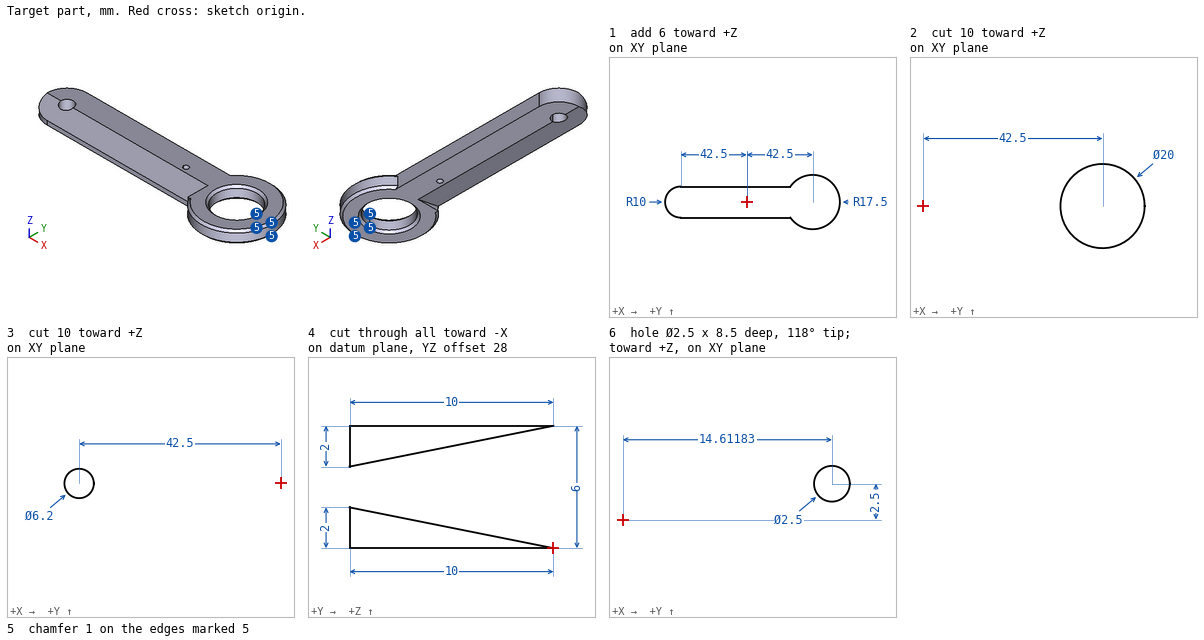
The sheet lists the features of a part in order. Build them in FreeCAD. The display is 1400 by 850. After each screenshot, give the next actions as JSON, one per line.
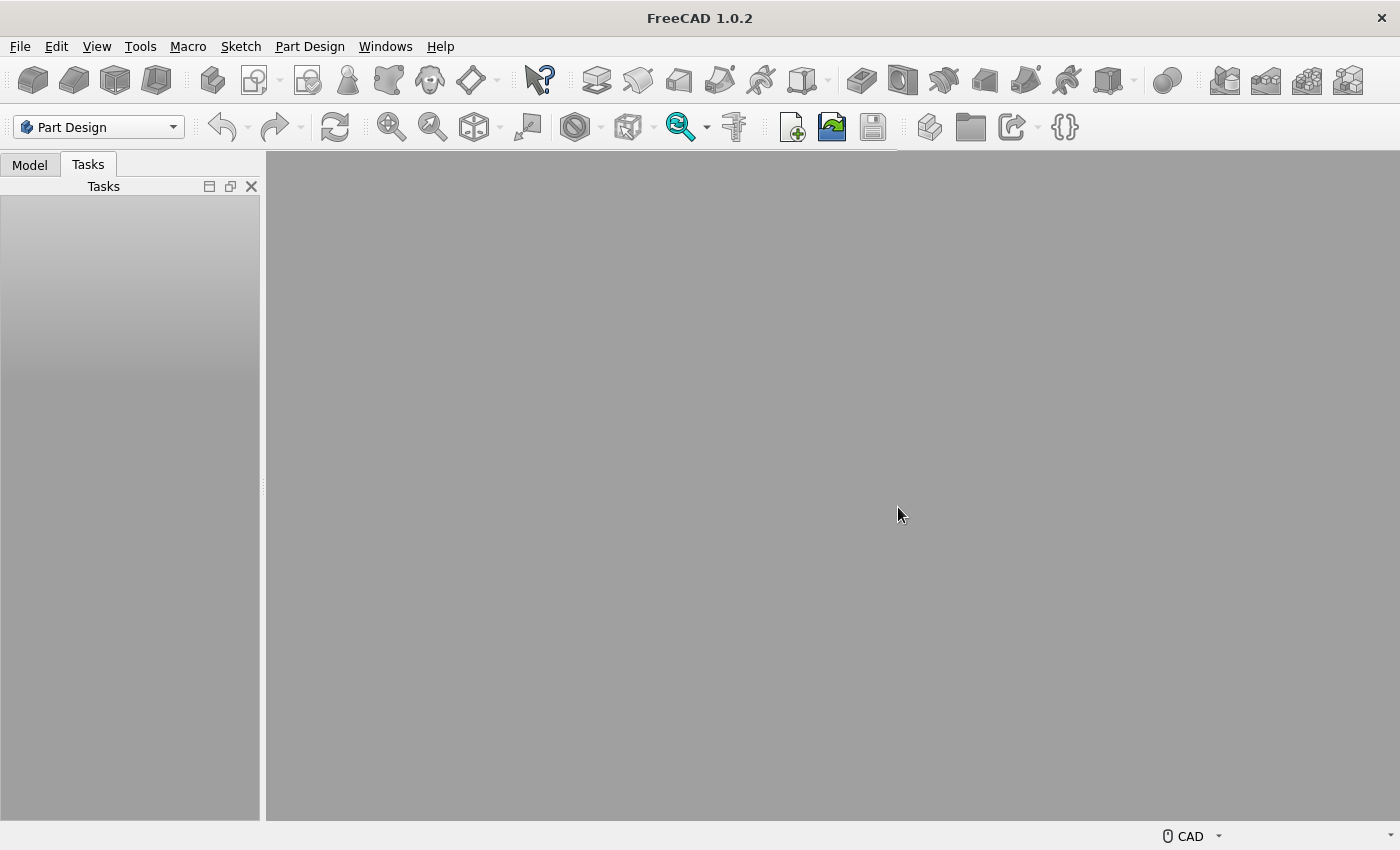
{"action": "key", "text": "ctrl+n"}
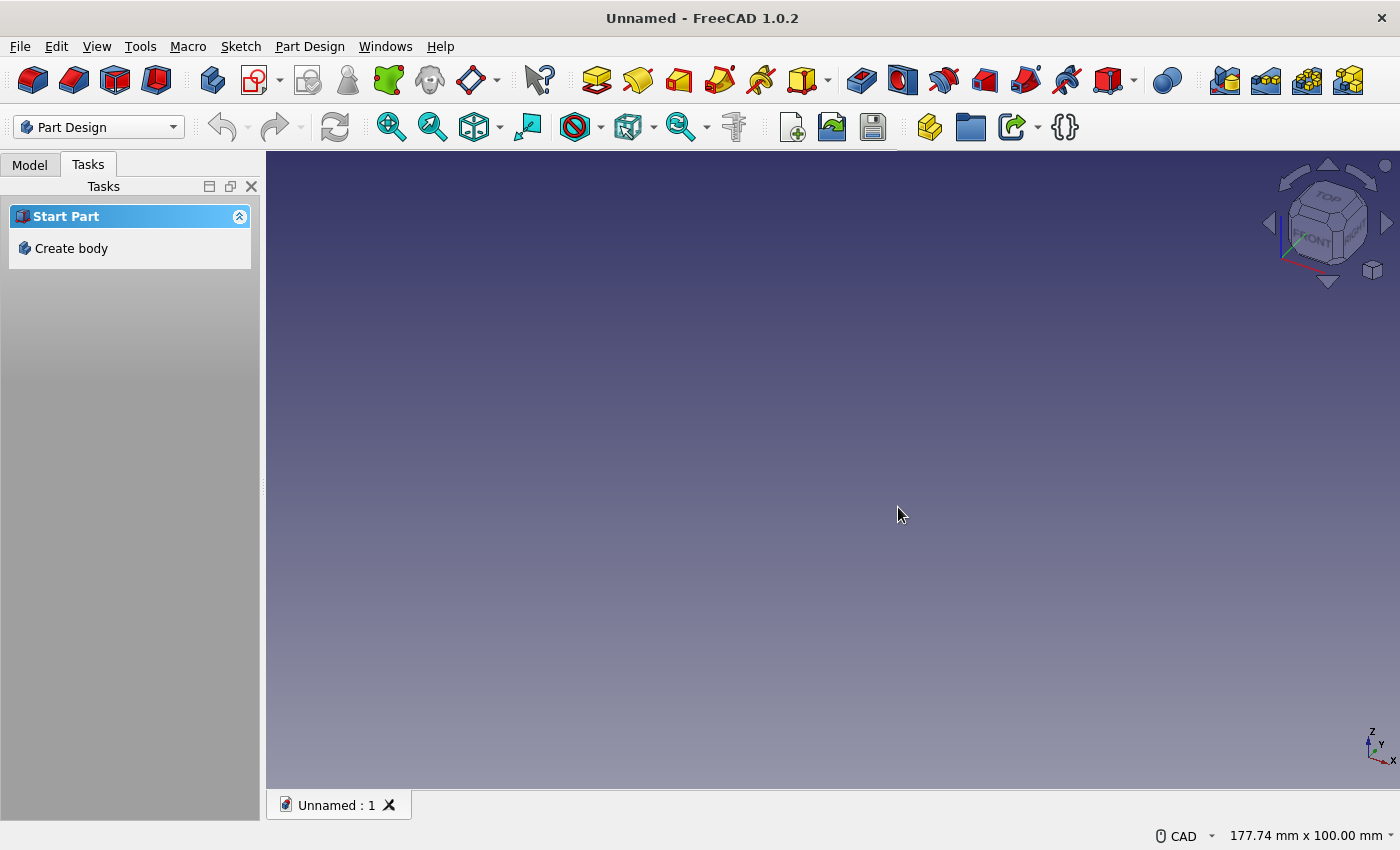
{"action": "left_click", "coordinate": [254, 80]}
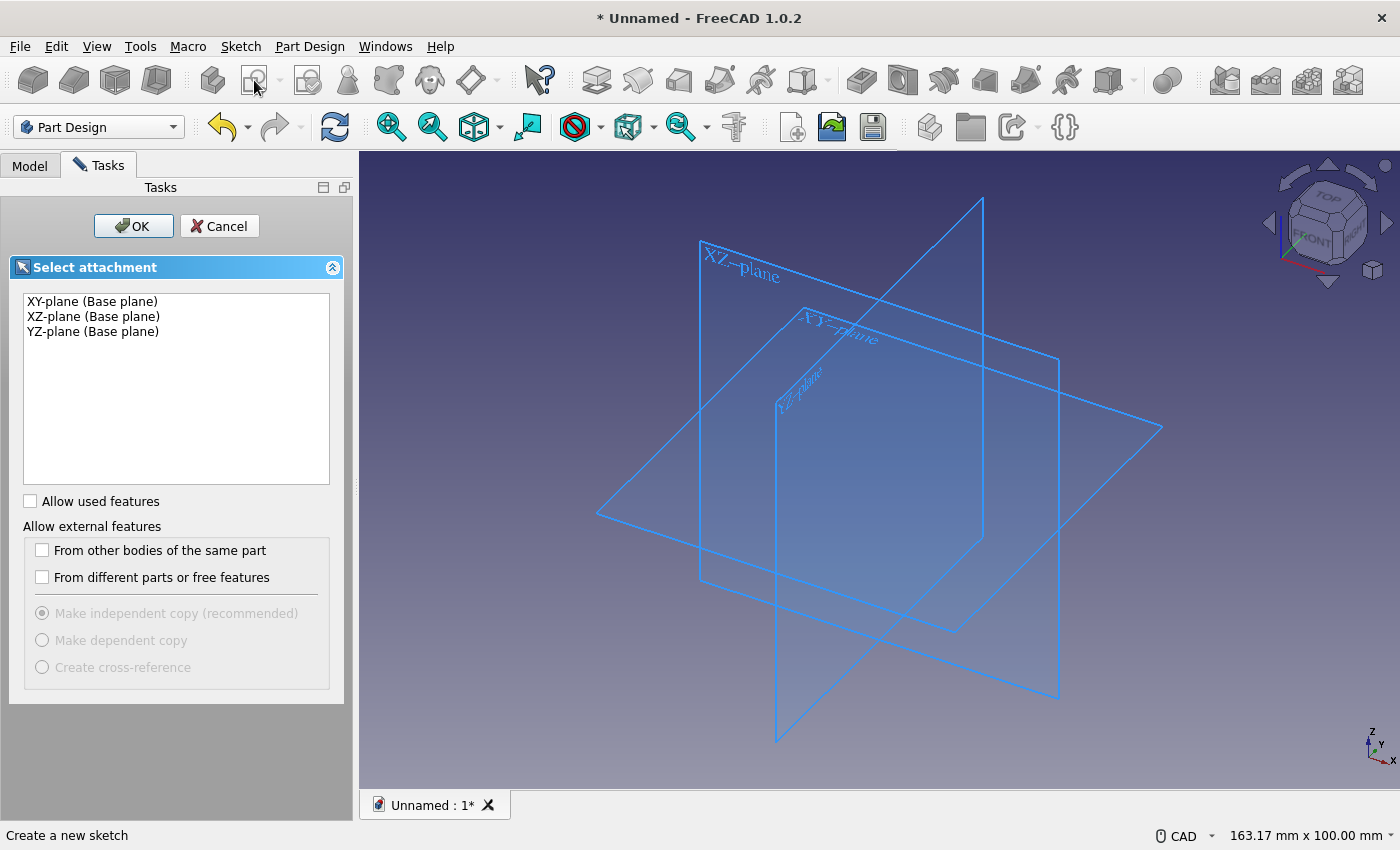
{"action": "left_click", "coordinate": [84, 302]}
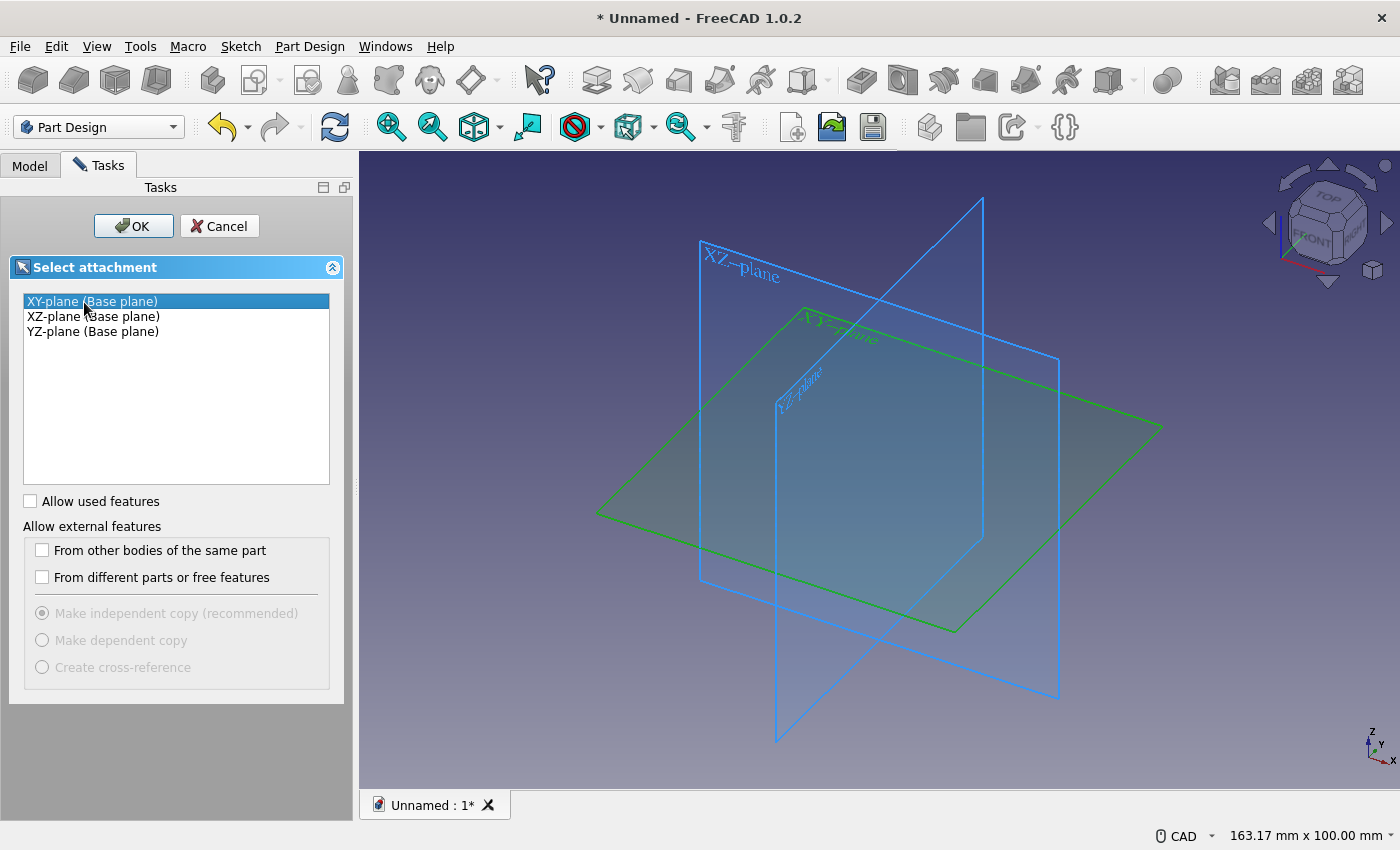
{"action": "left_click", "coordinate": [134, 226]}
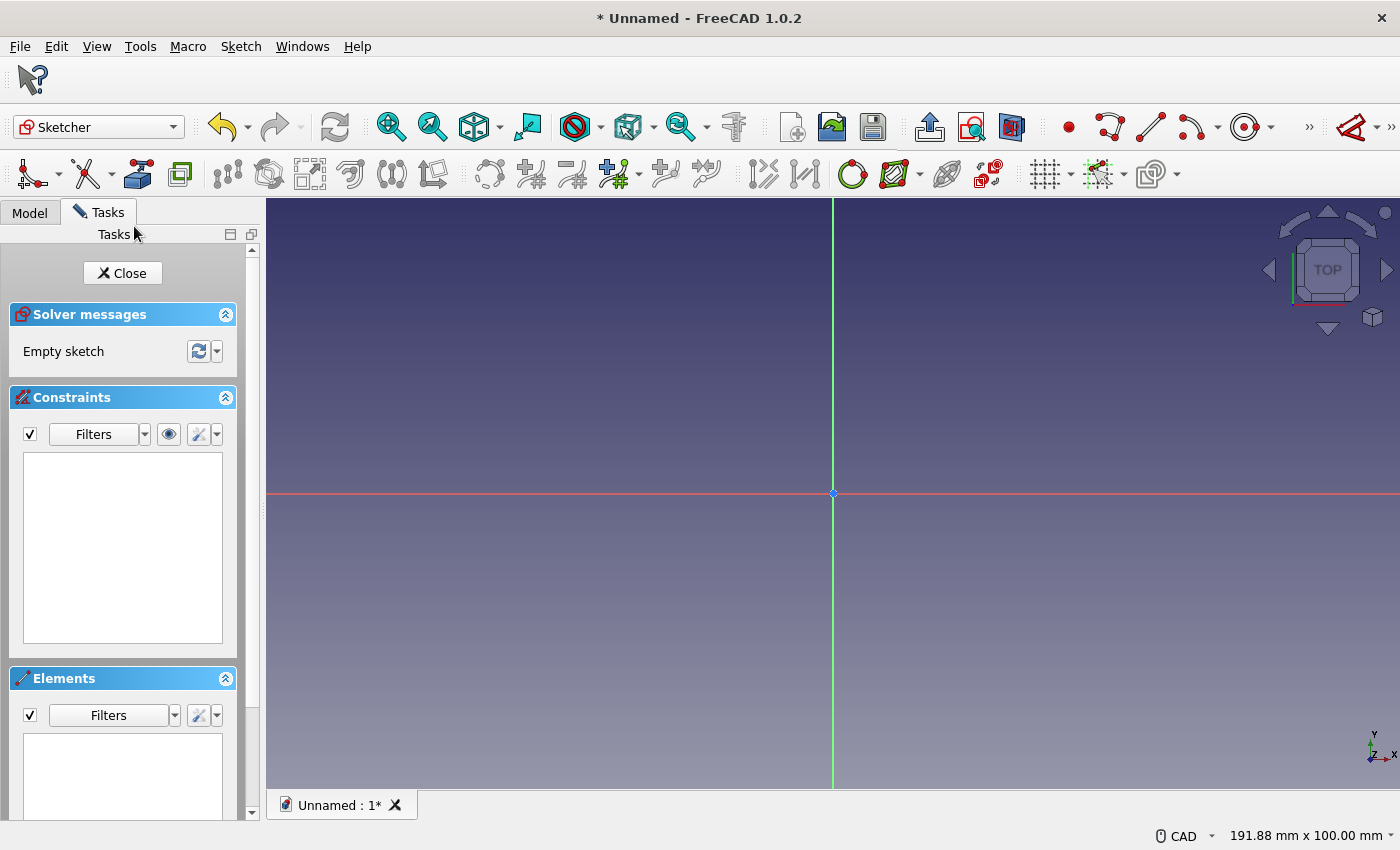
{"action": "key", "text": "g l"}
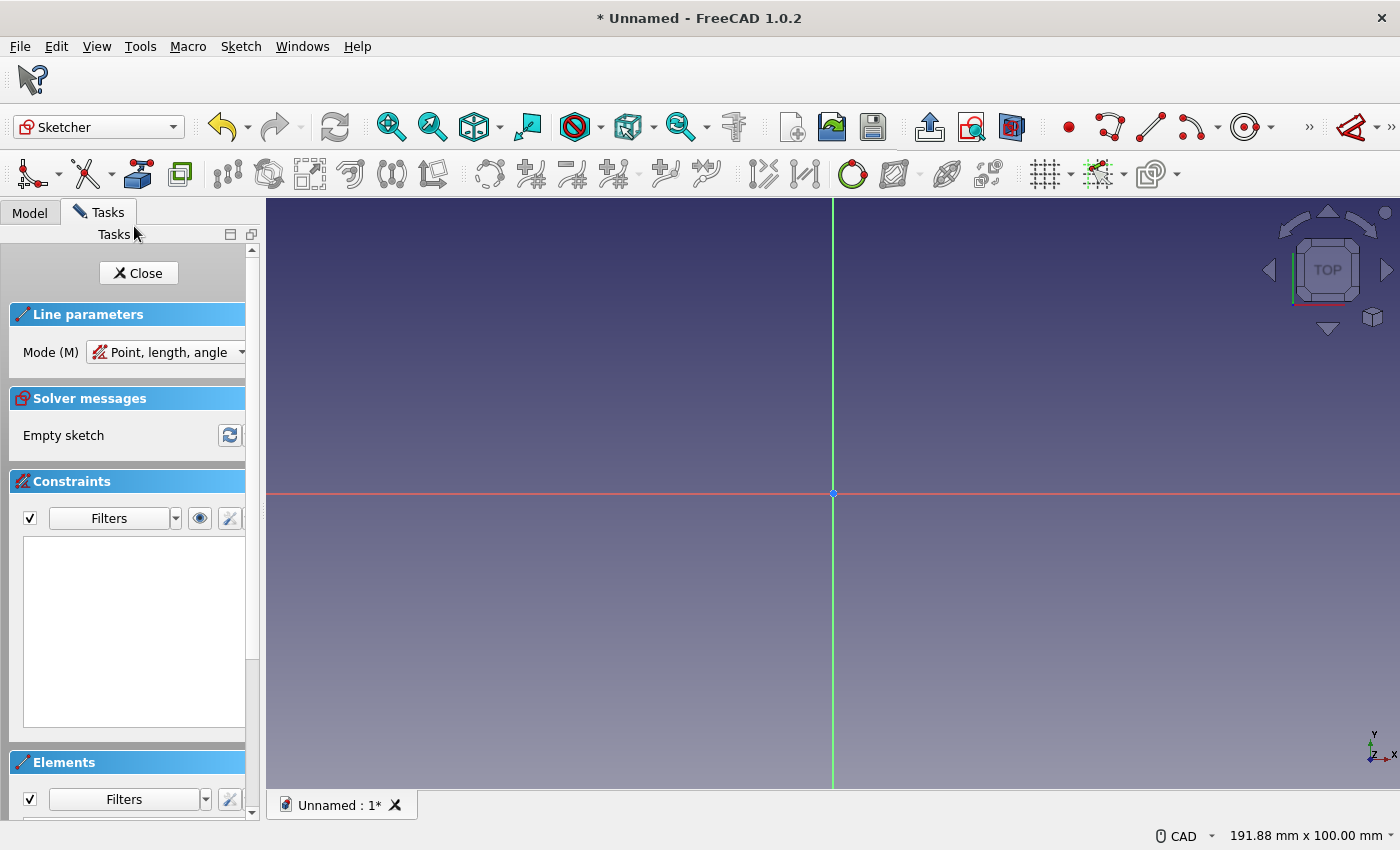
{"action": "left_click", "coordinate": [999, 434]}
{"action": "left_click", "coordinate": [582, 434]}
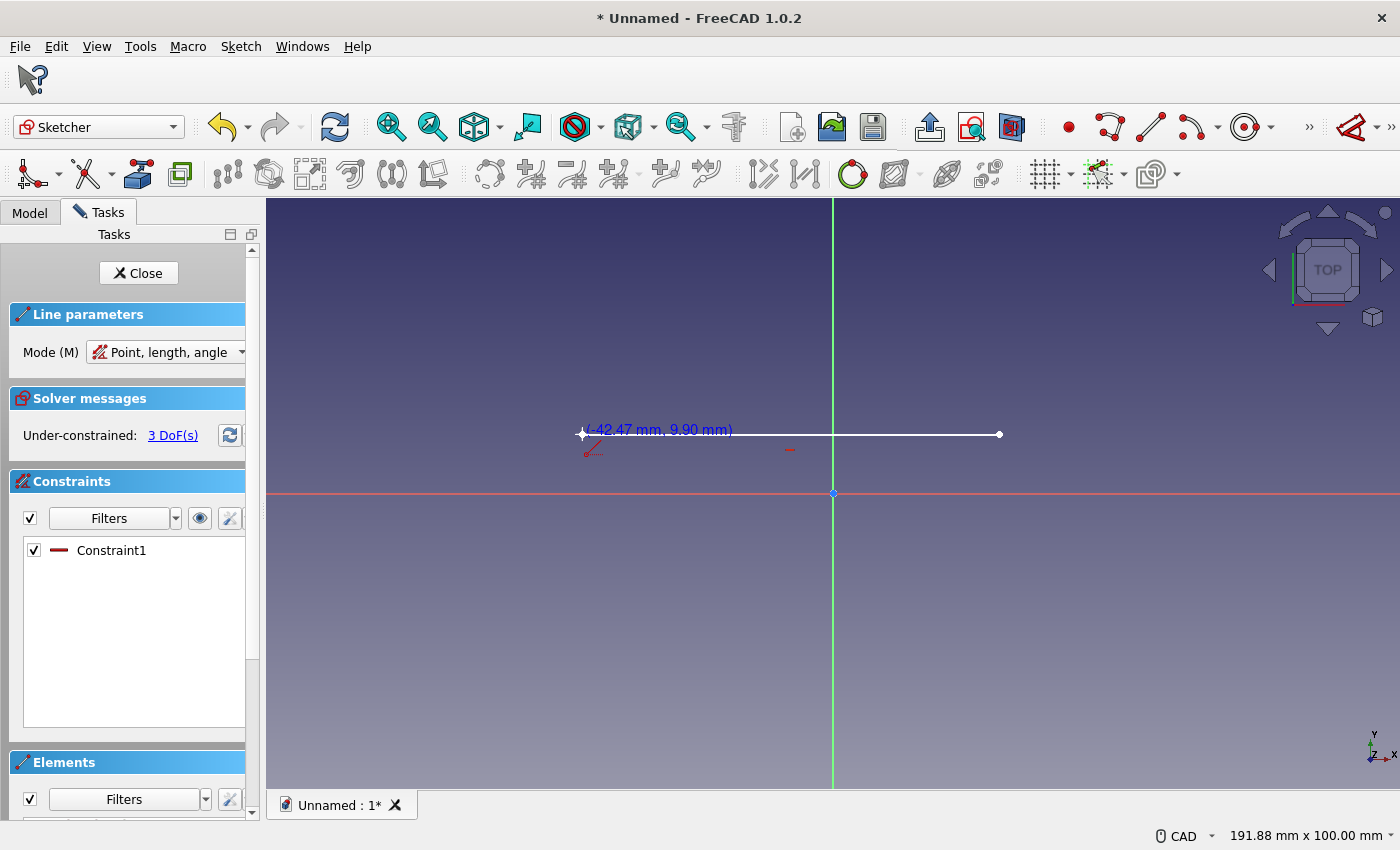
{"action": "left_click", "coordinate": [582, 553]}
{"action": "left_click", "coordinate": [999, 553]}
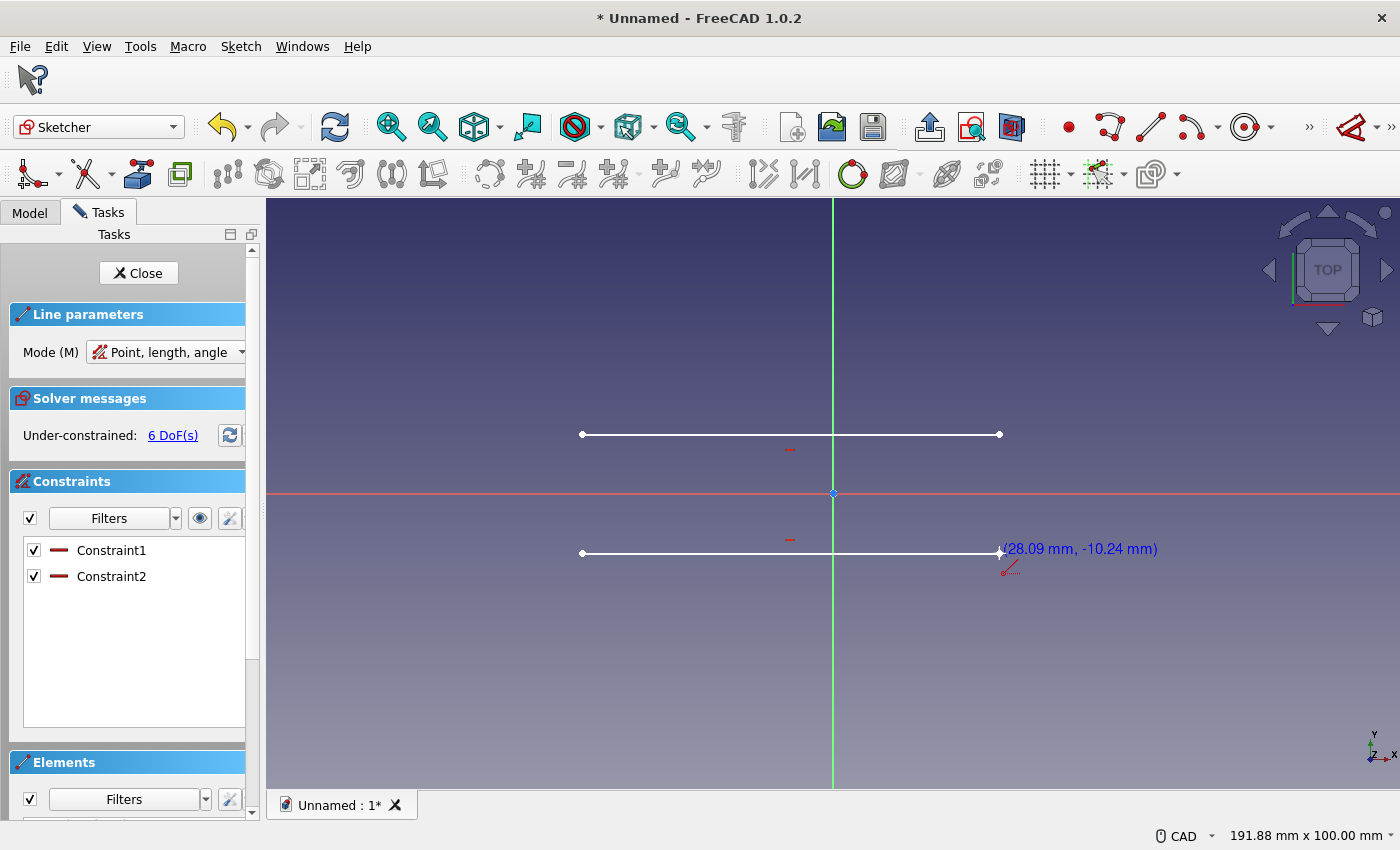
{"action": "key", "text": "g 3 a"}